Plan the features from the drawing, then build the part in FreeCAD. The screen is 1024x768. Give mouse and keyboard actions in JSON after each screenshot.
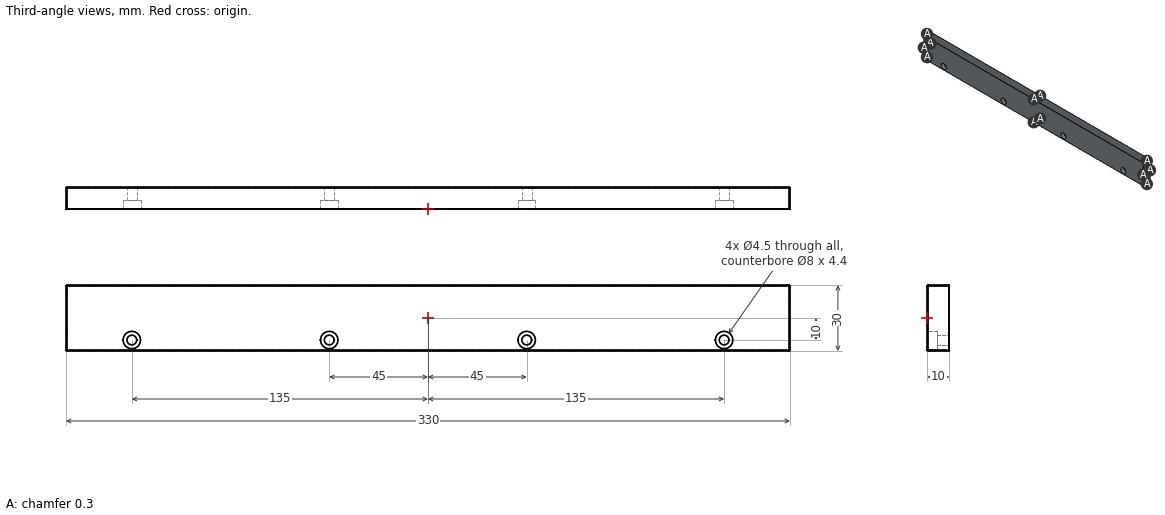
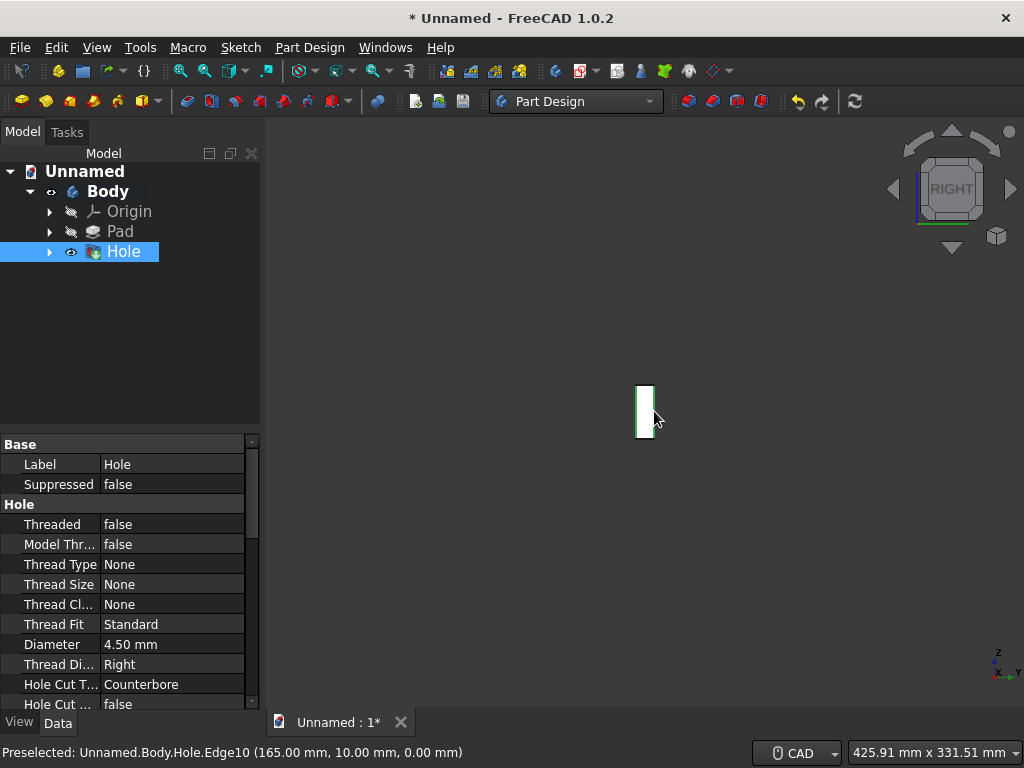
{"action": "key", "text": "5"}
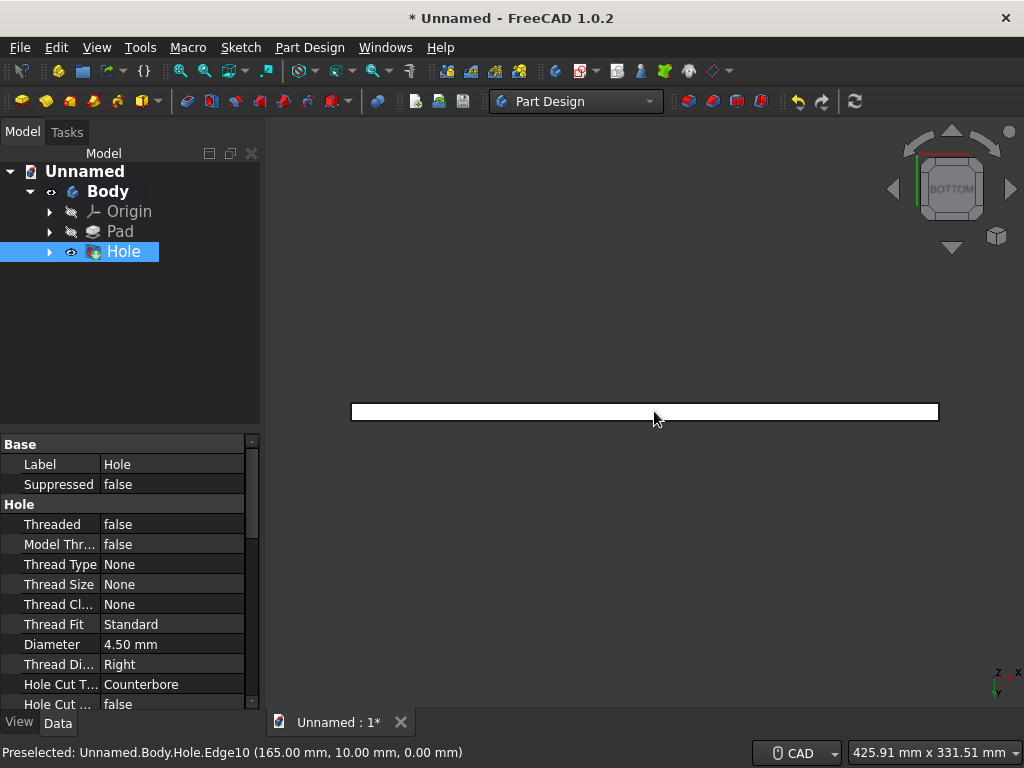
{"action": "left_click", "coordinate": [897, 411], "text": "ctrl"}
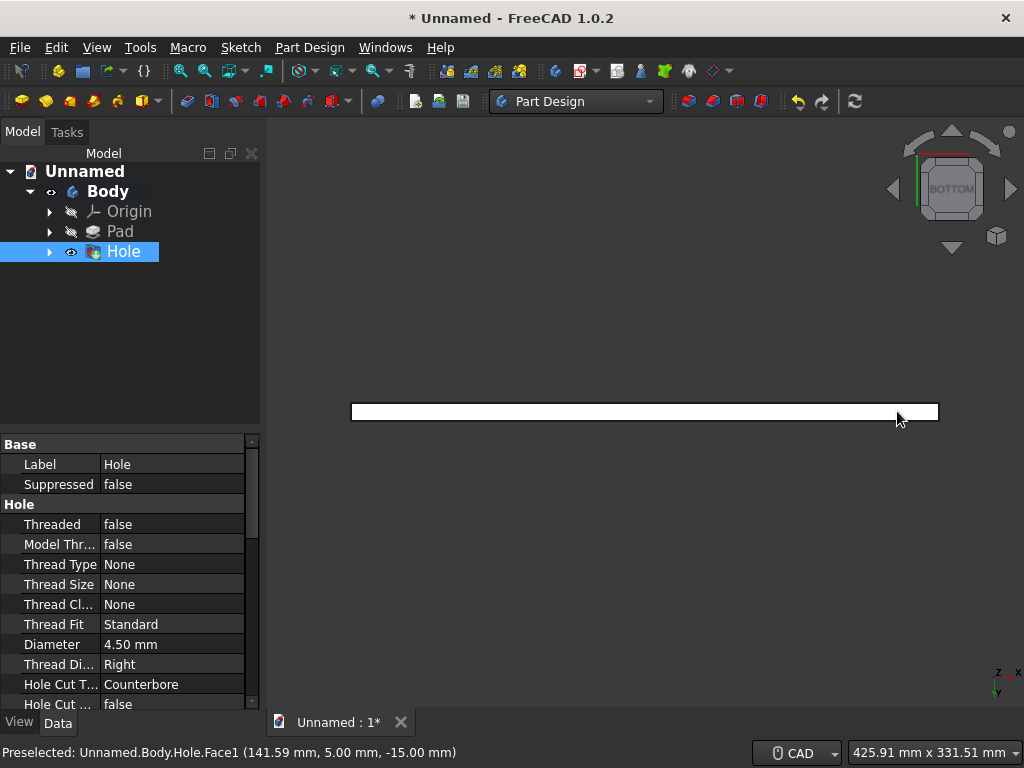
{"action": "key", "text": "4"}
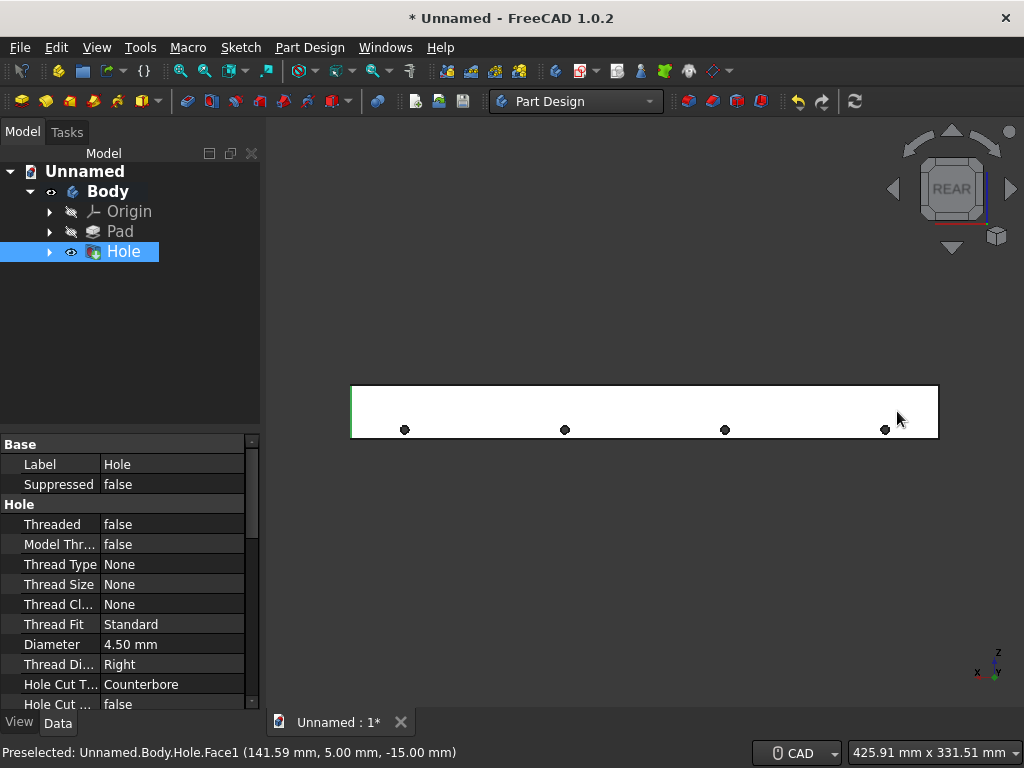
{"action": "left_click", "coordinate": [939, 411], "text": "ctrl"}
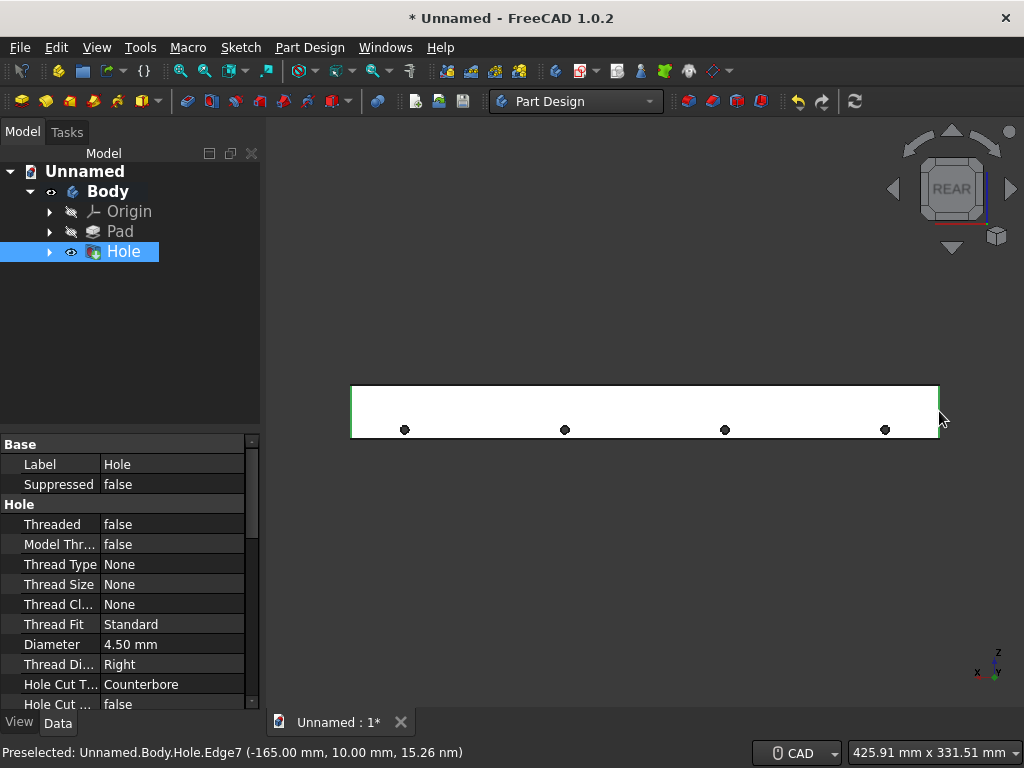
{"action": "left_click", "coordinate": [714, 102]}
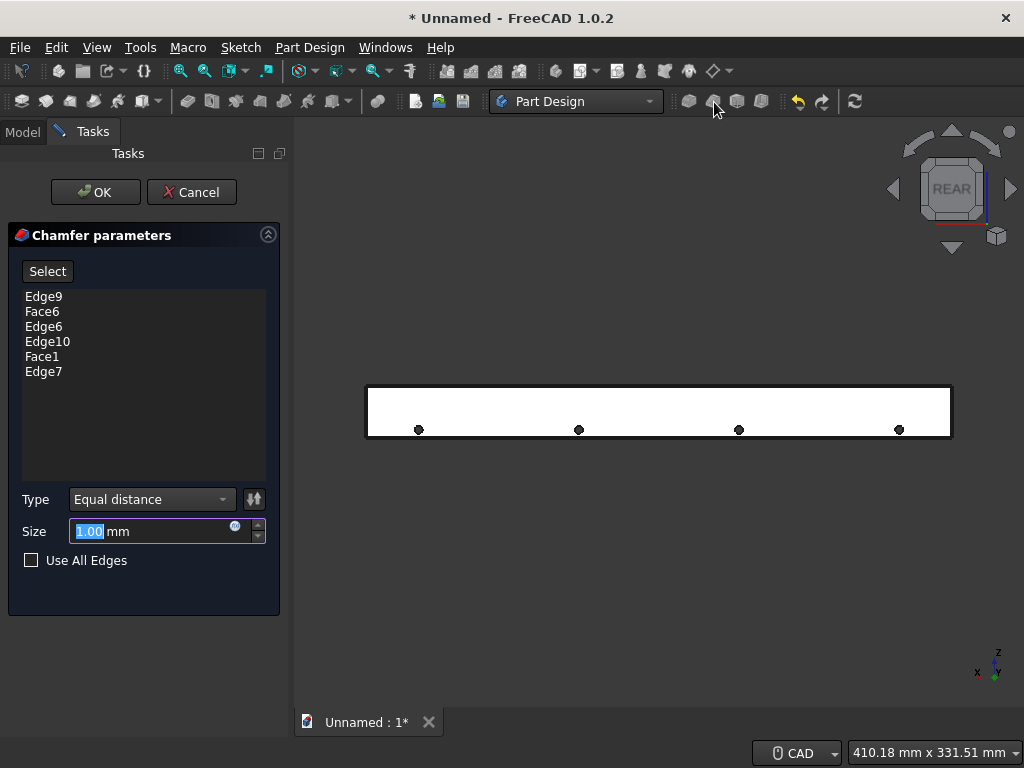
{"action": "type", "text": "0.3"}
{"action": "key", "text": "Tab"}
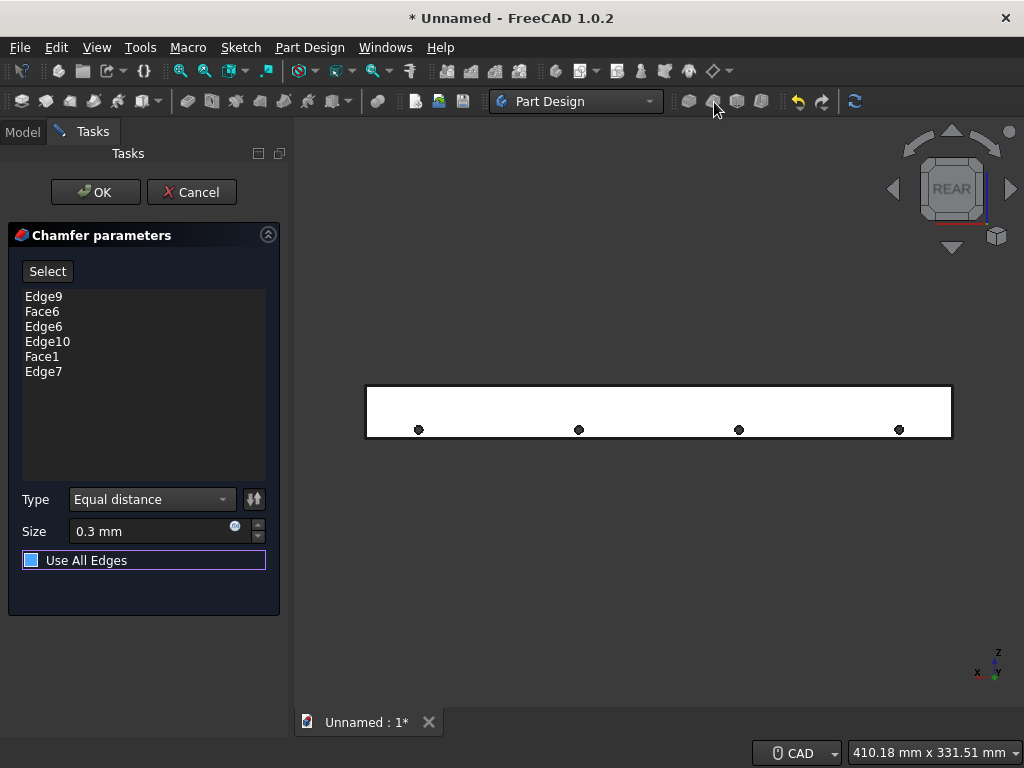
{"action": "left_click", "coordinate": [96, 192]}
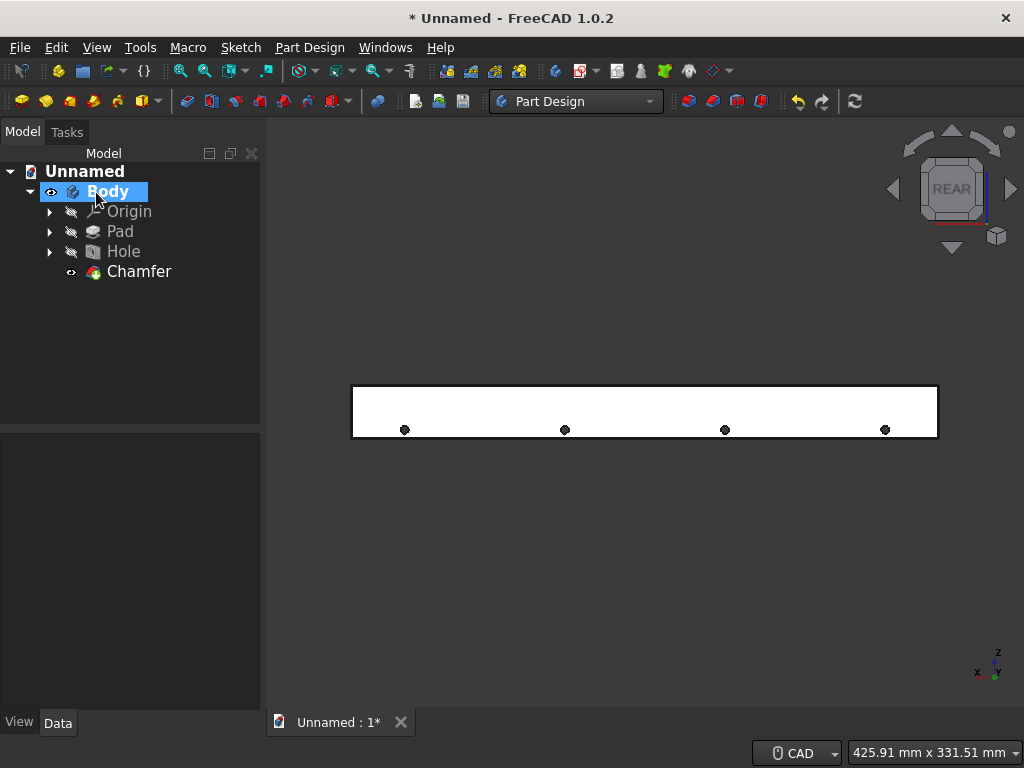
{"action": "key", "text": "0"}